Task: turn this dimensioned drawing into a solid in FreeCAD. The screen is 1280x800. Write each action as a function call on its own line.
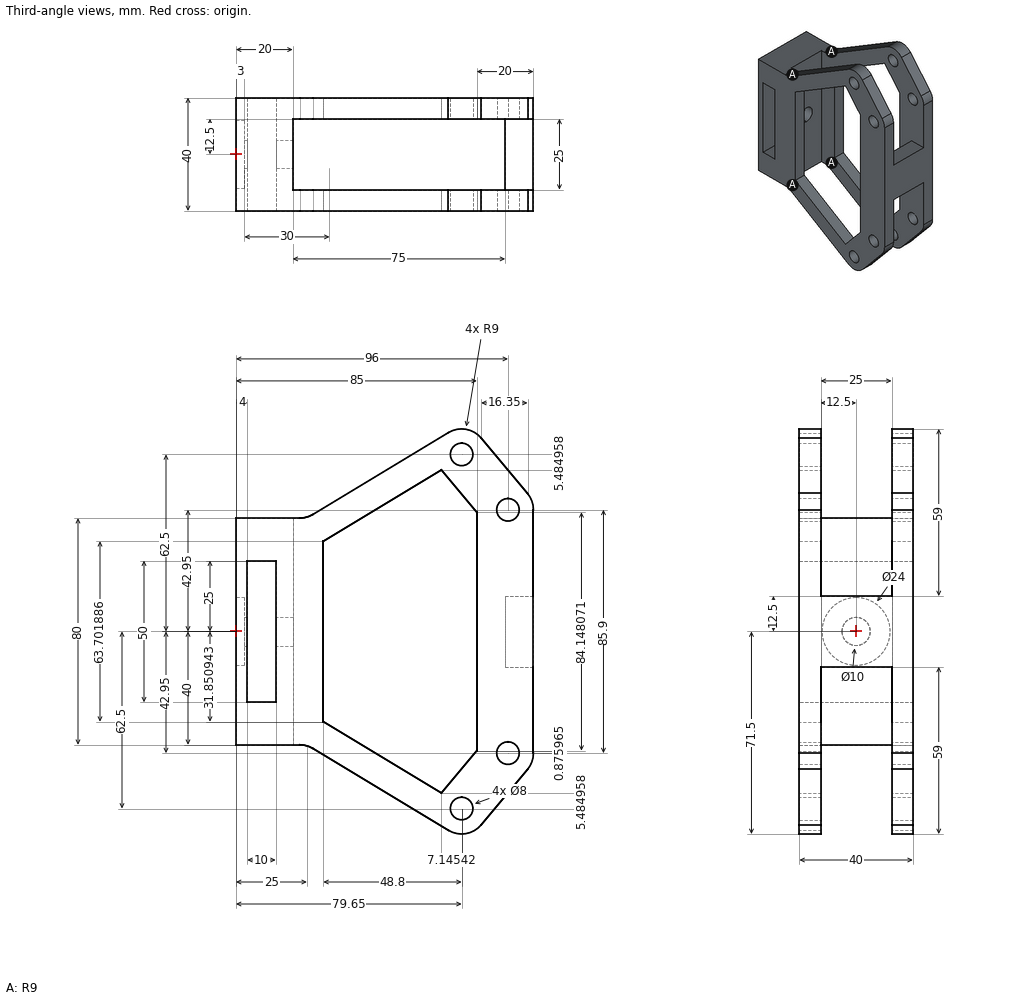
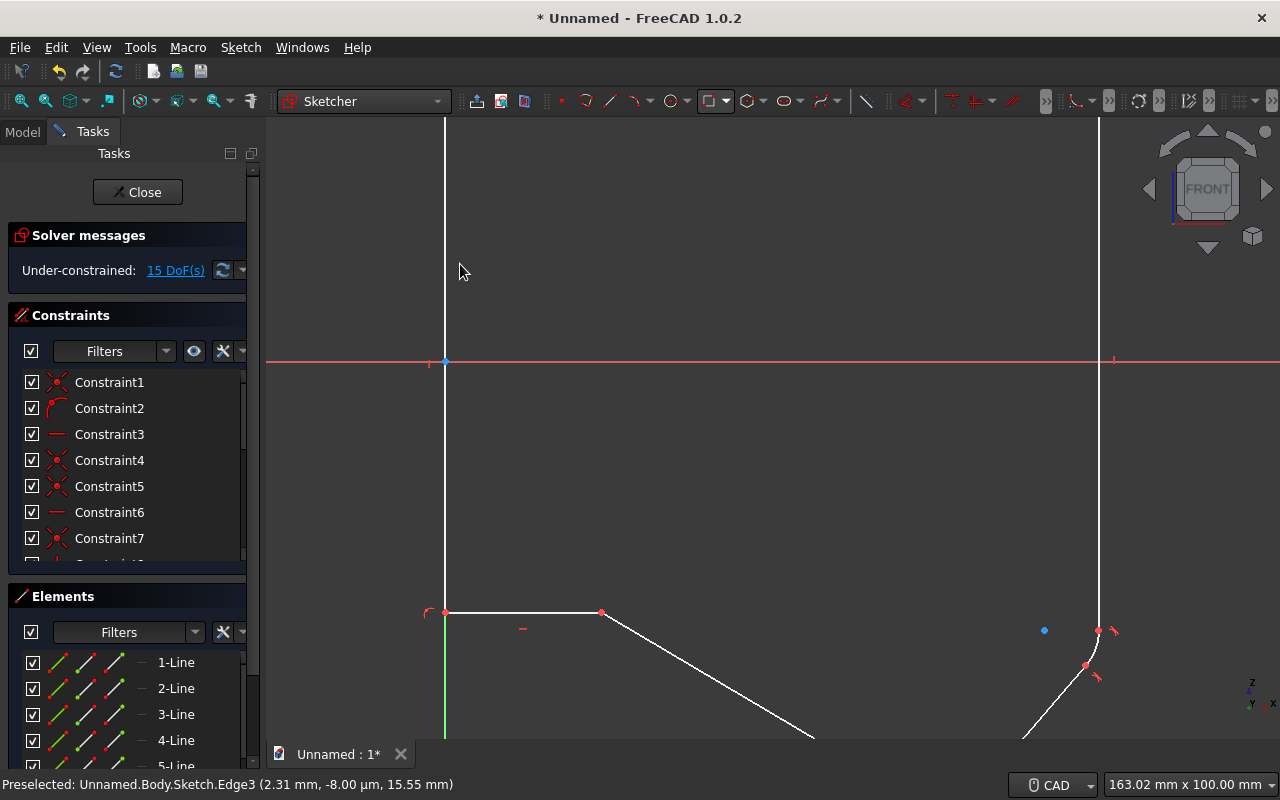
scroll(650, 482, down, 4)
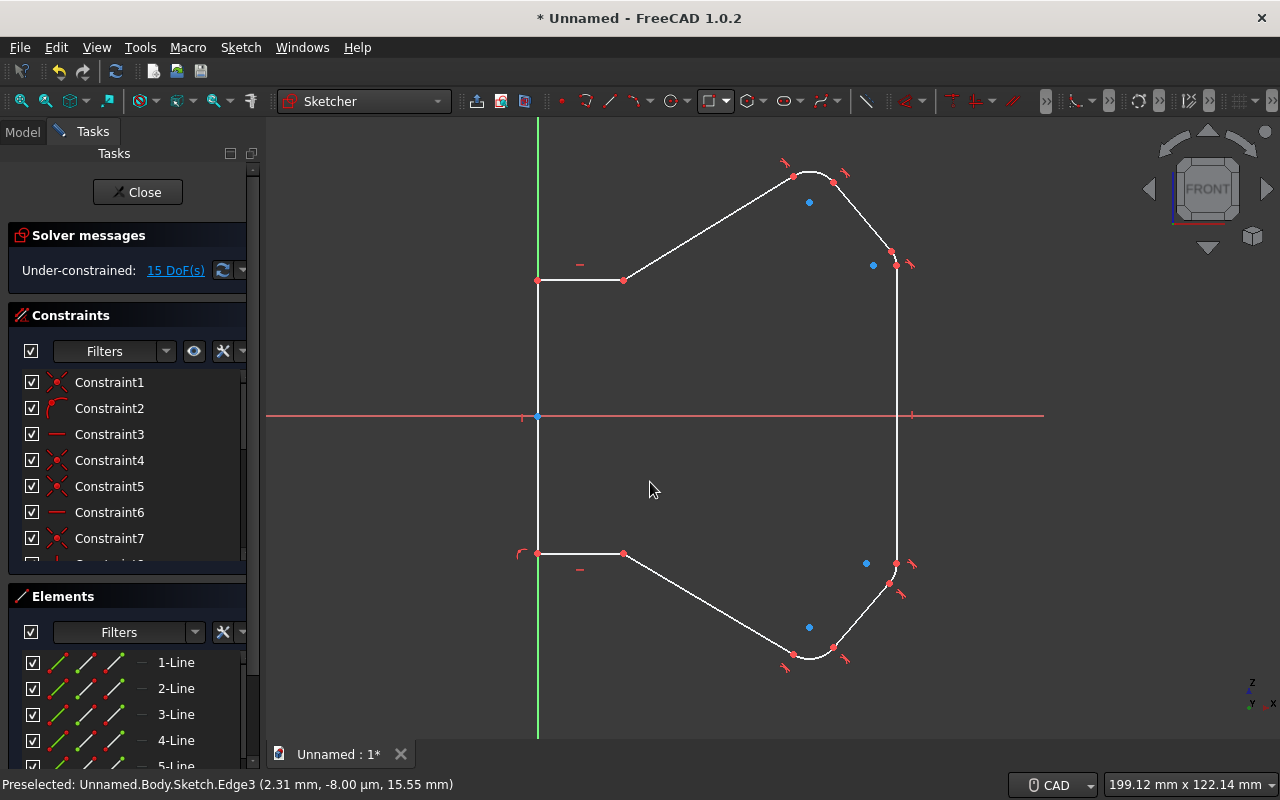
scroll(792, 230, up, 2)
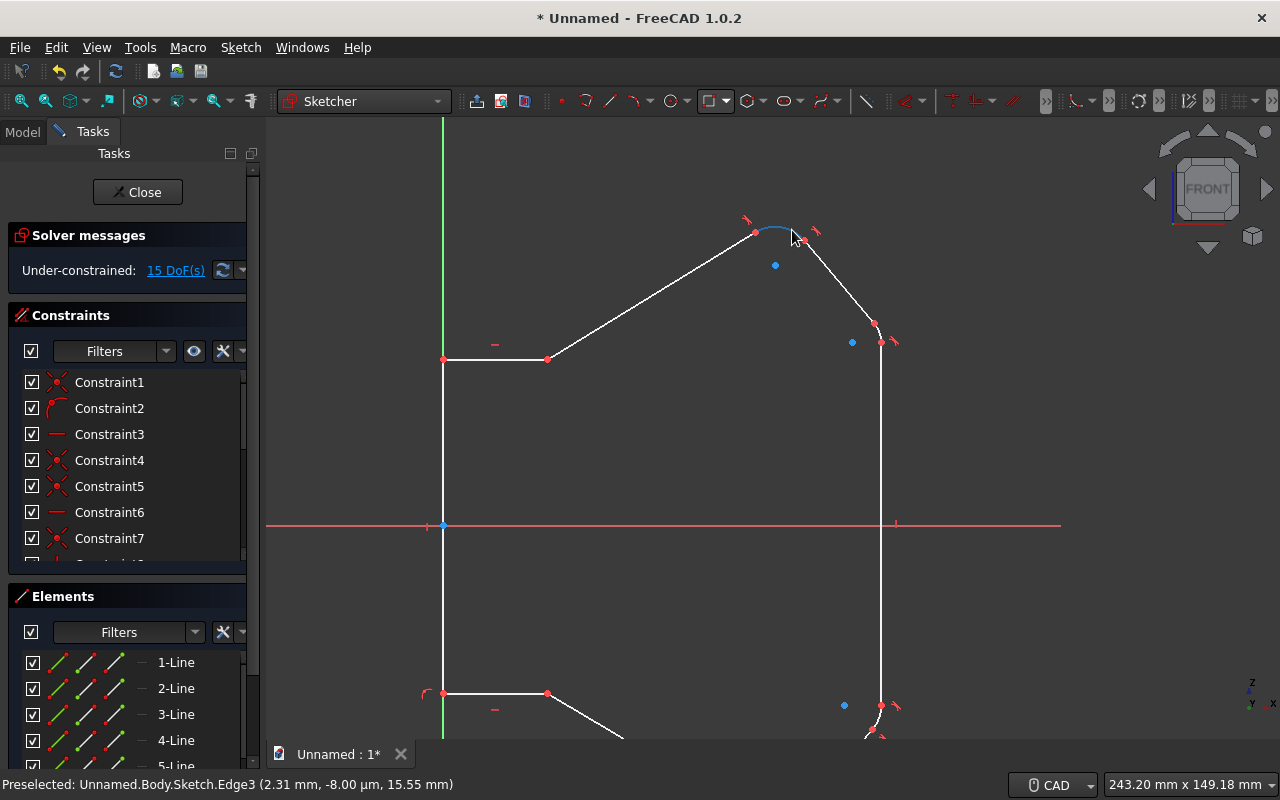
click(792, 231)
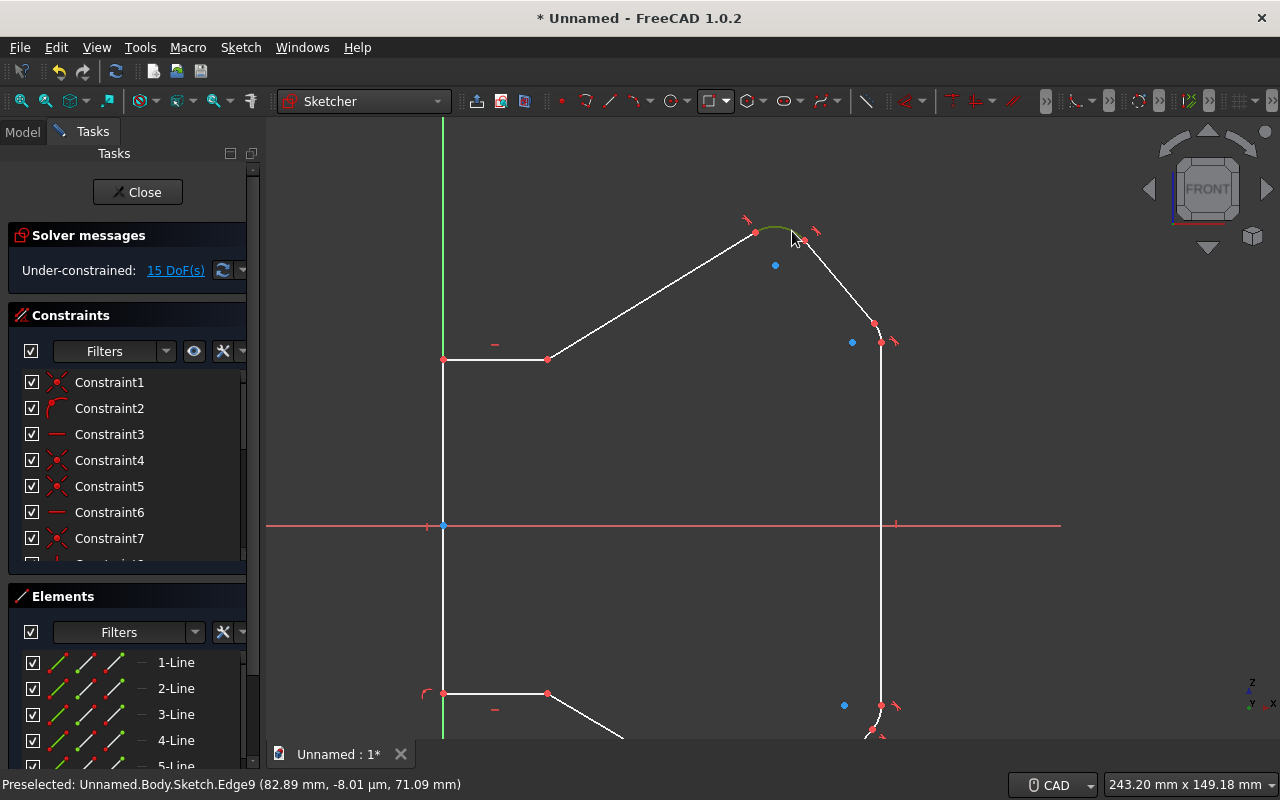
scroll(879, 332, up, 2)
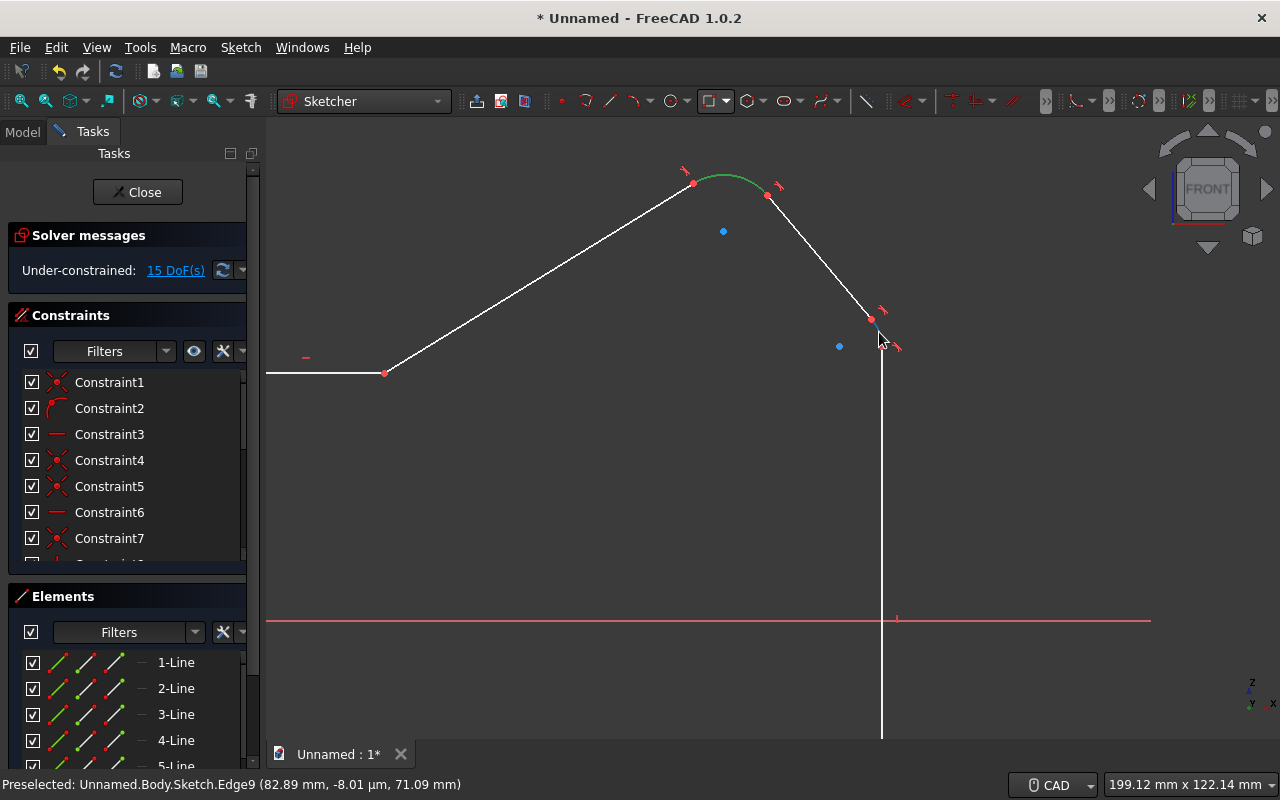
click(879, 332)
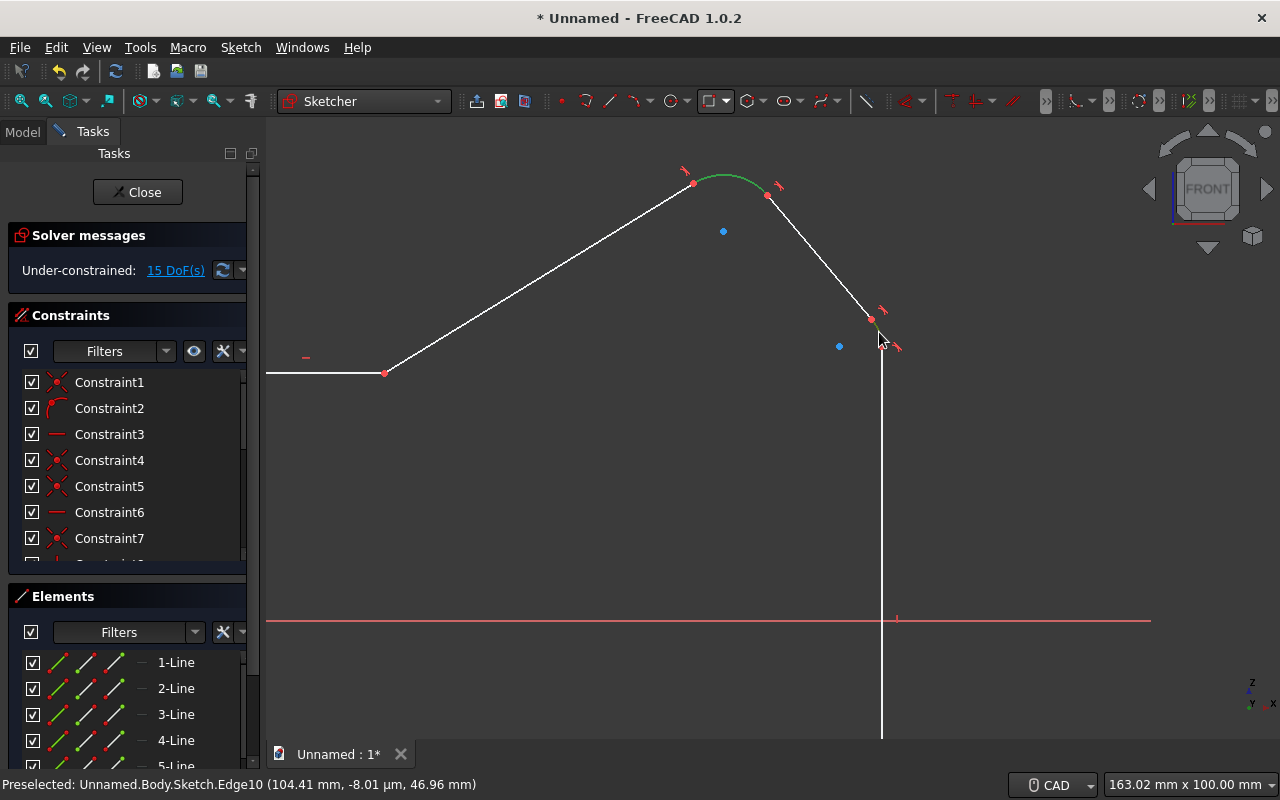
scroll(827, 271, down, 4)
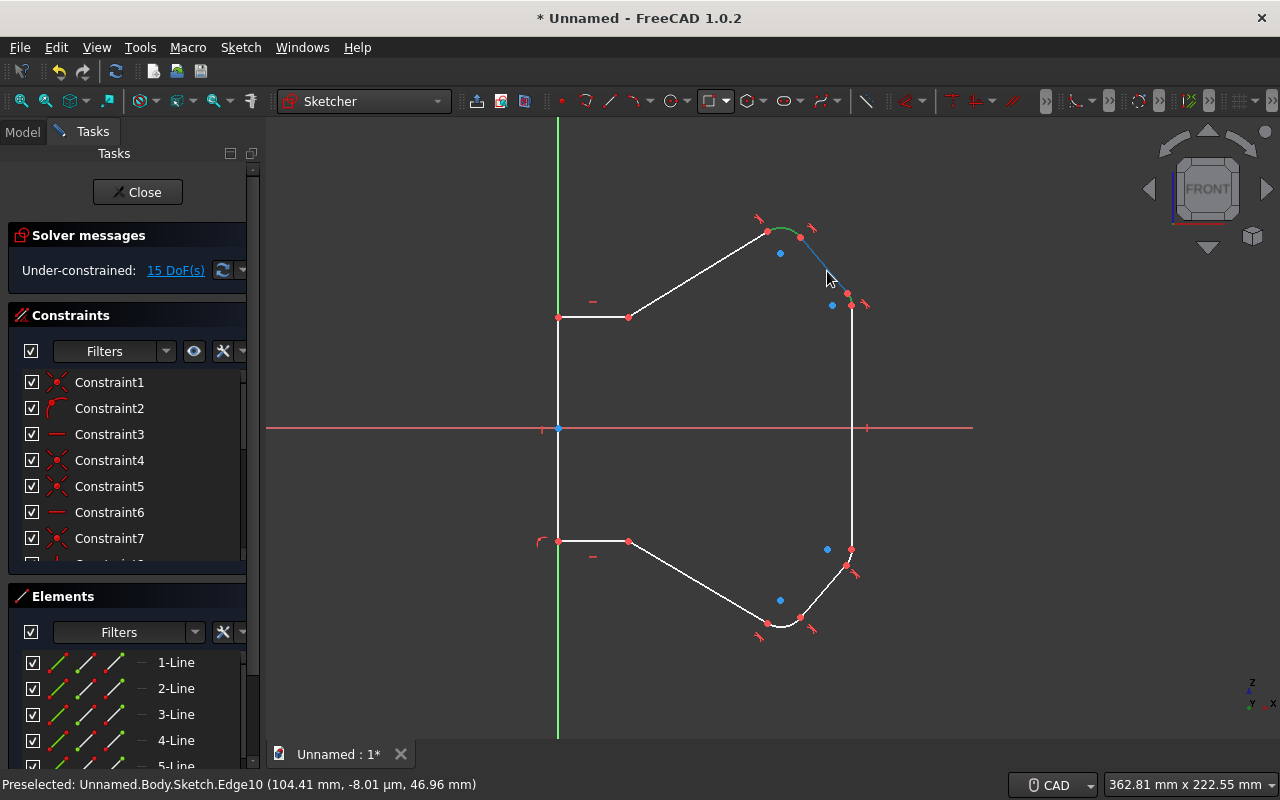
scroll(849, 561, up, 5)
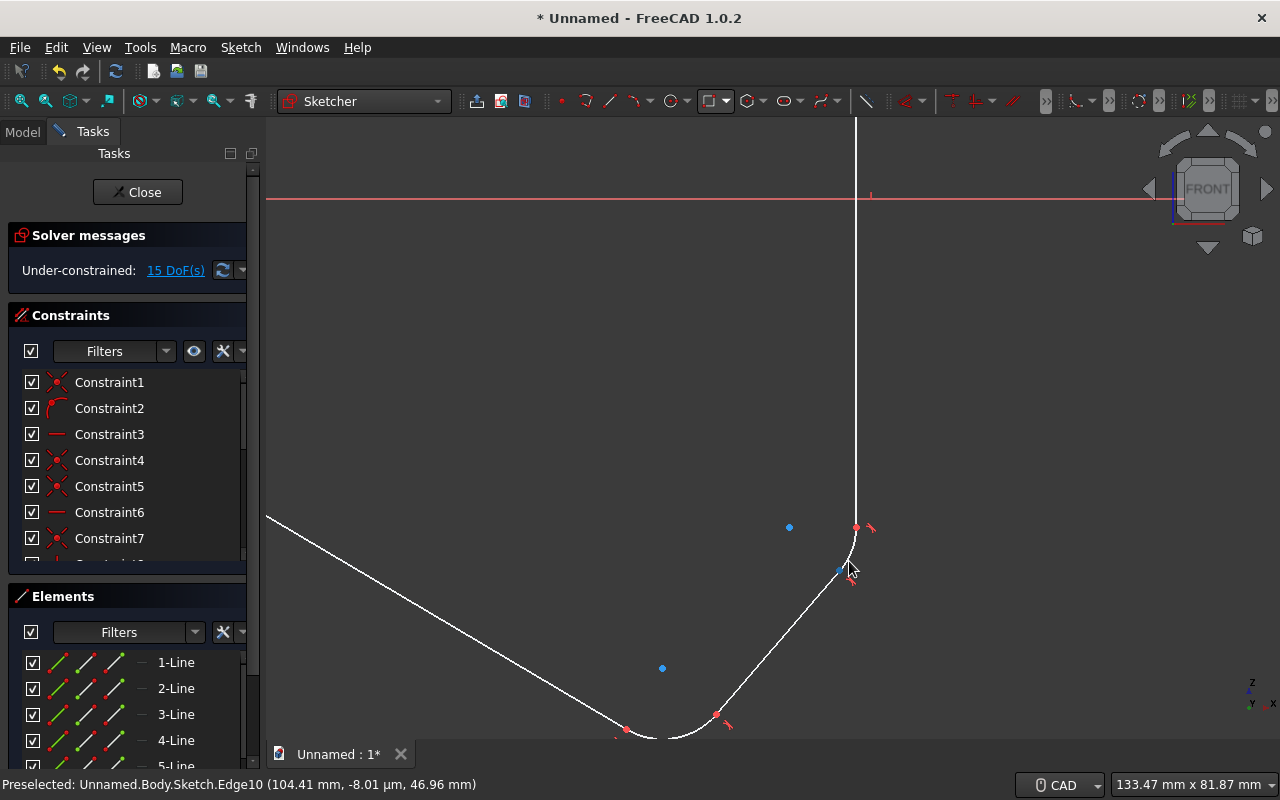
click(848, 559)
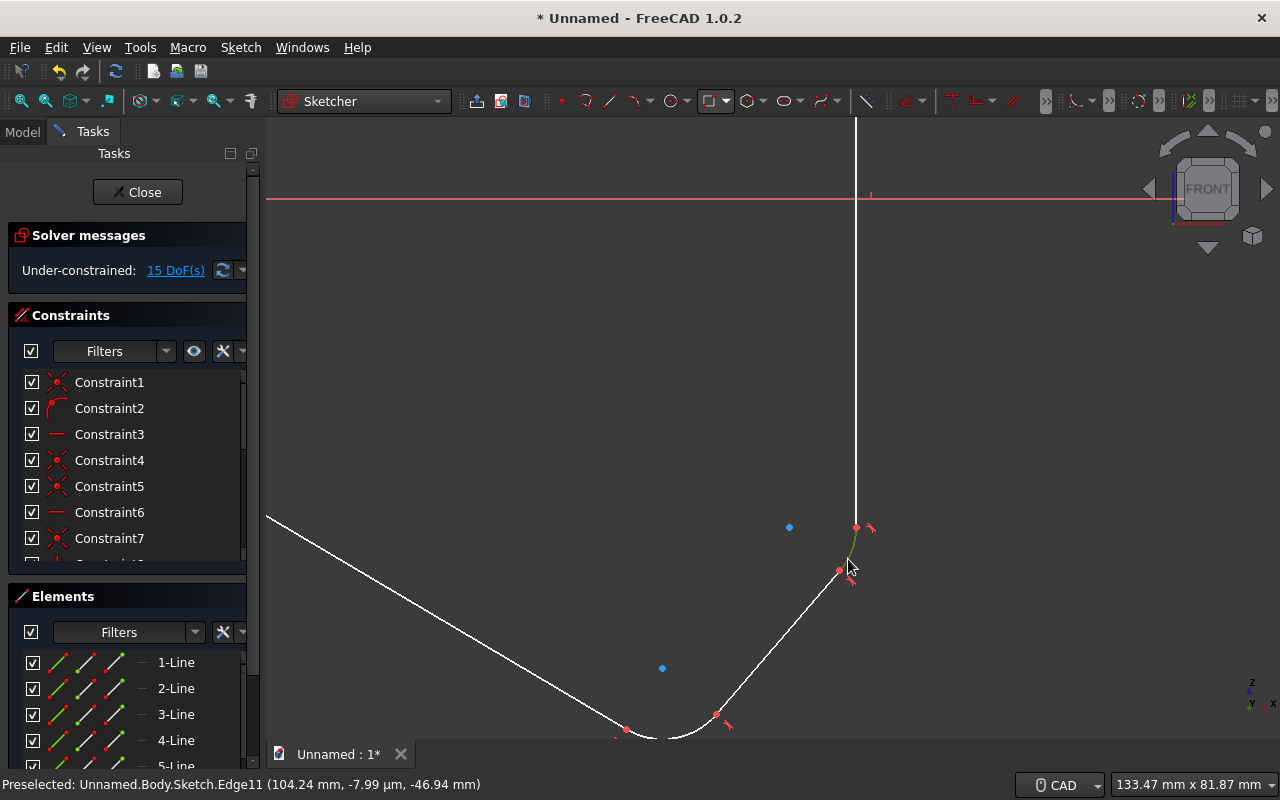
scroll(849, 561, down, 5)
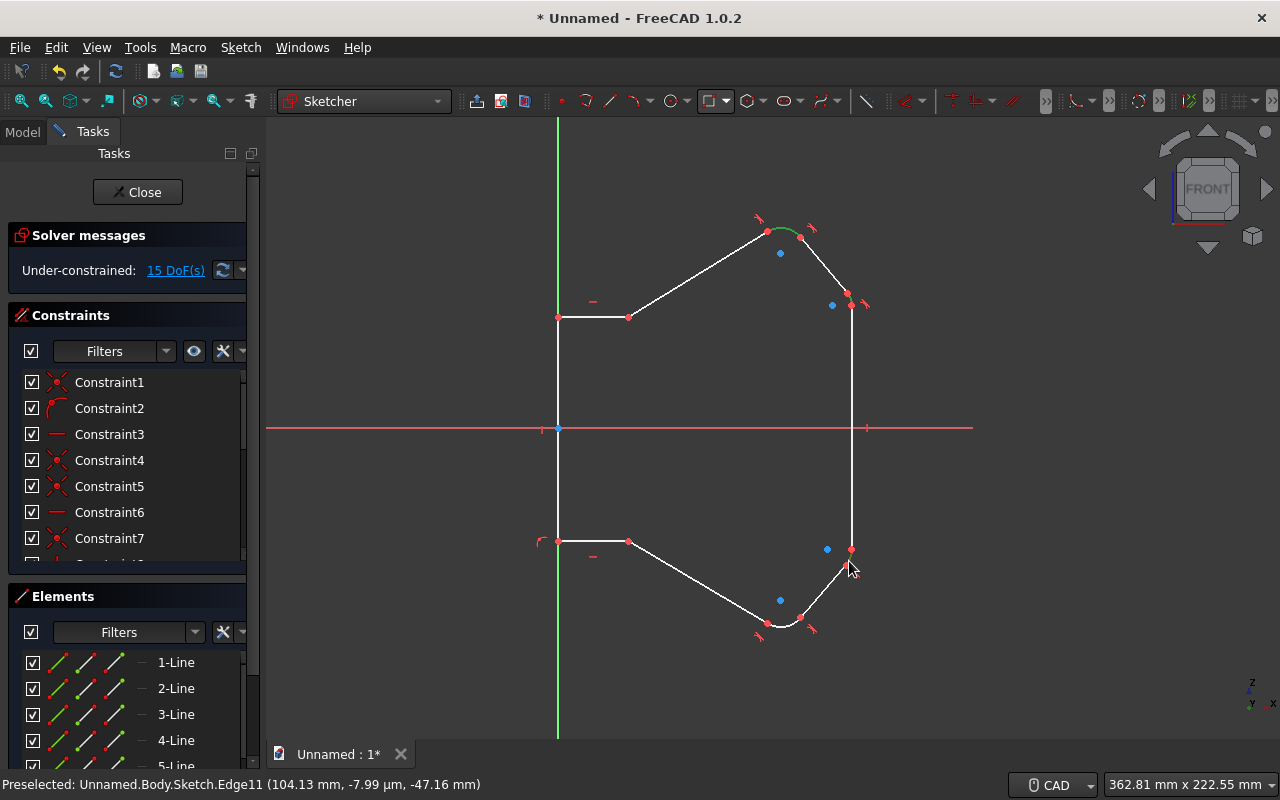
scroll(778, 627, up, 2)